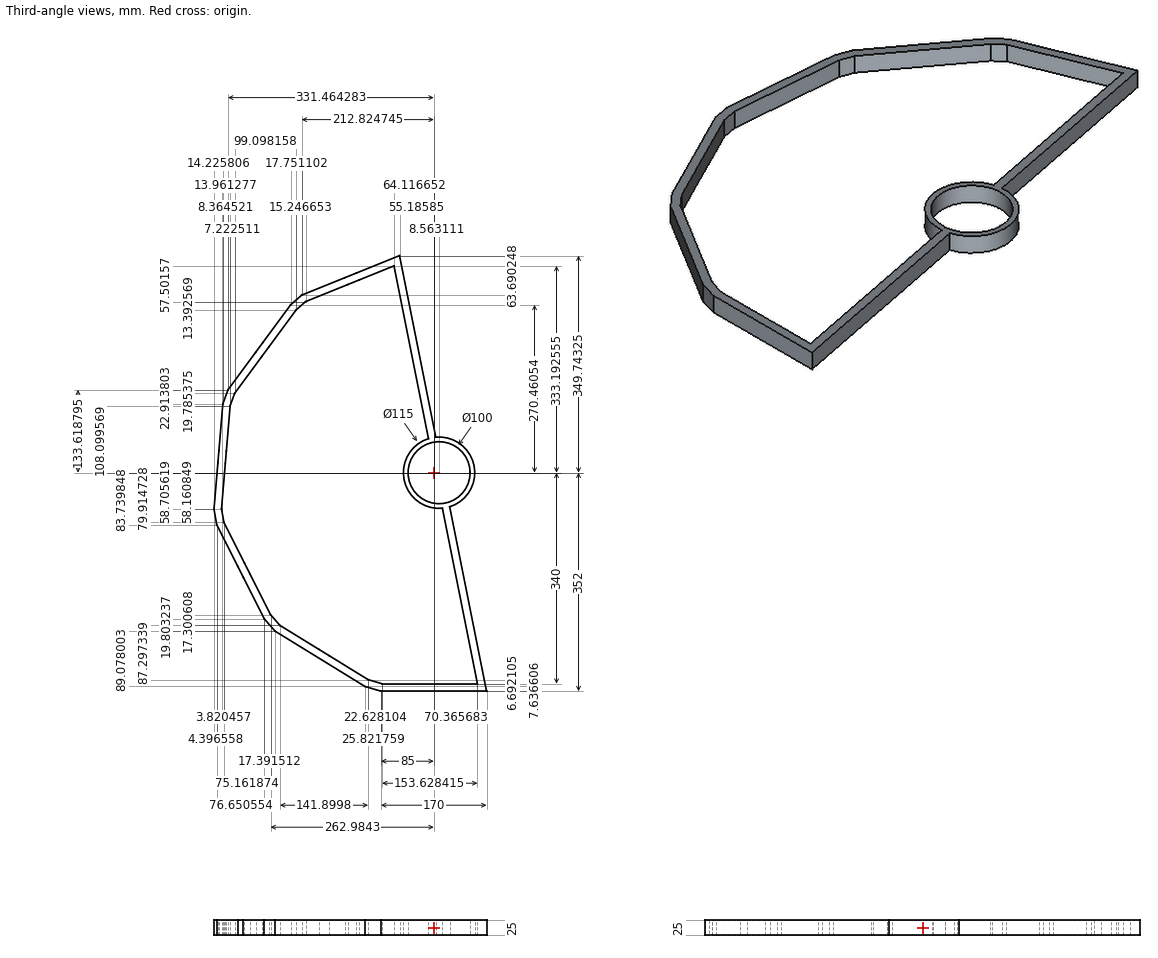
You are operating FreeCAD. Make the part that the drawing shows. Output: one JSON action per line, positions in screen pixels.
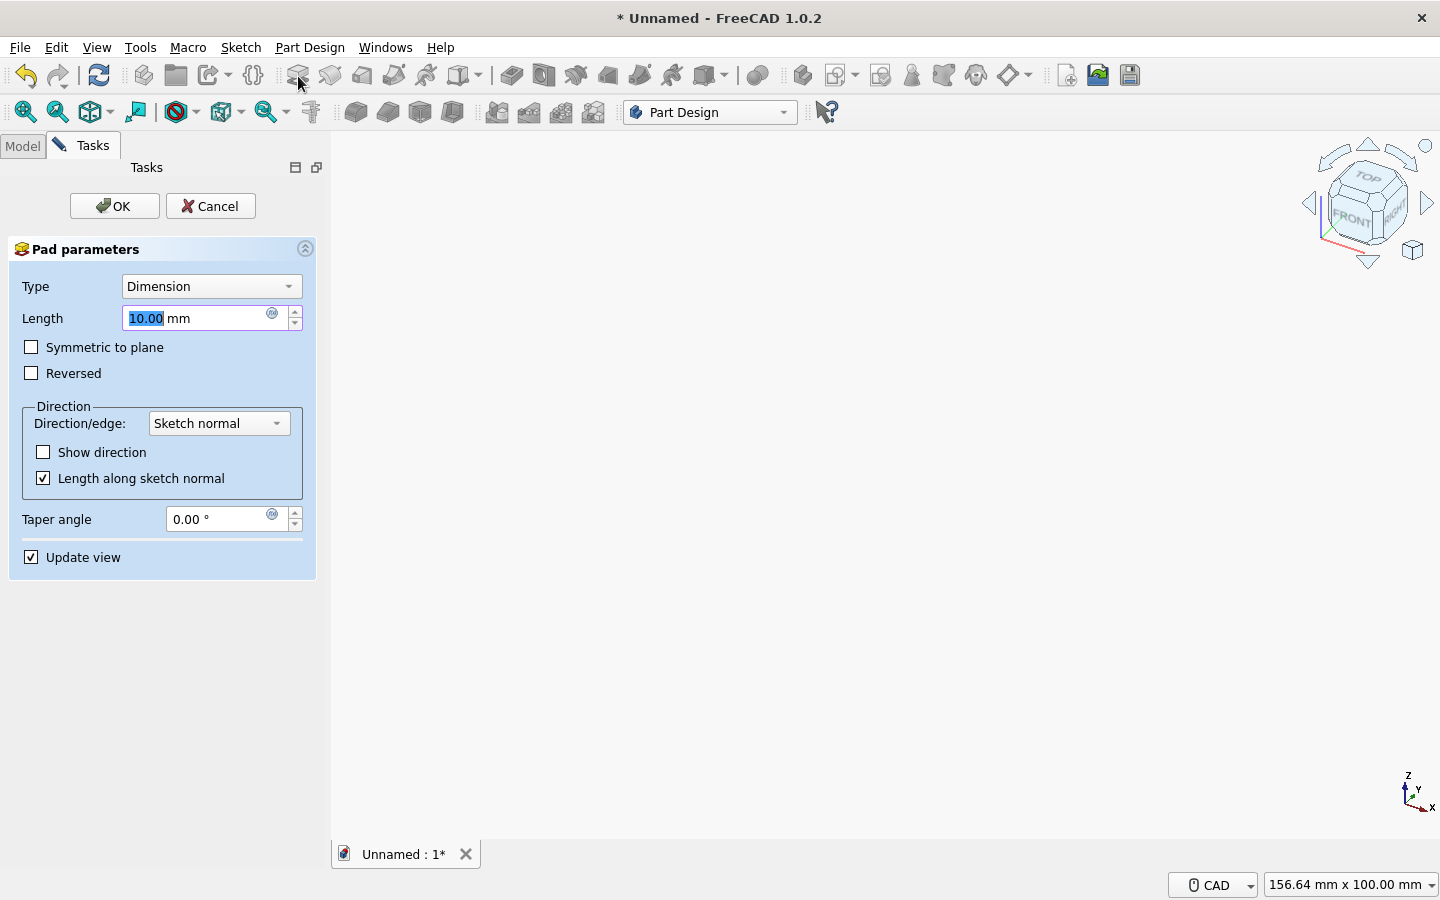
{"action": "type", "text": "25"}
{"action": "key", "text": "Tab"}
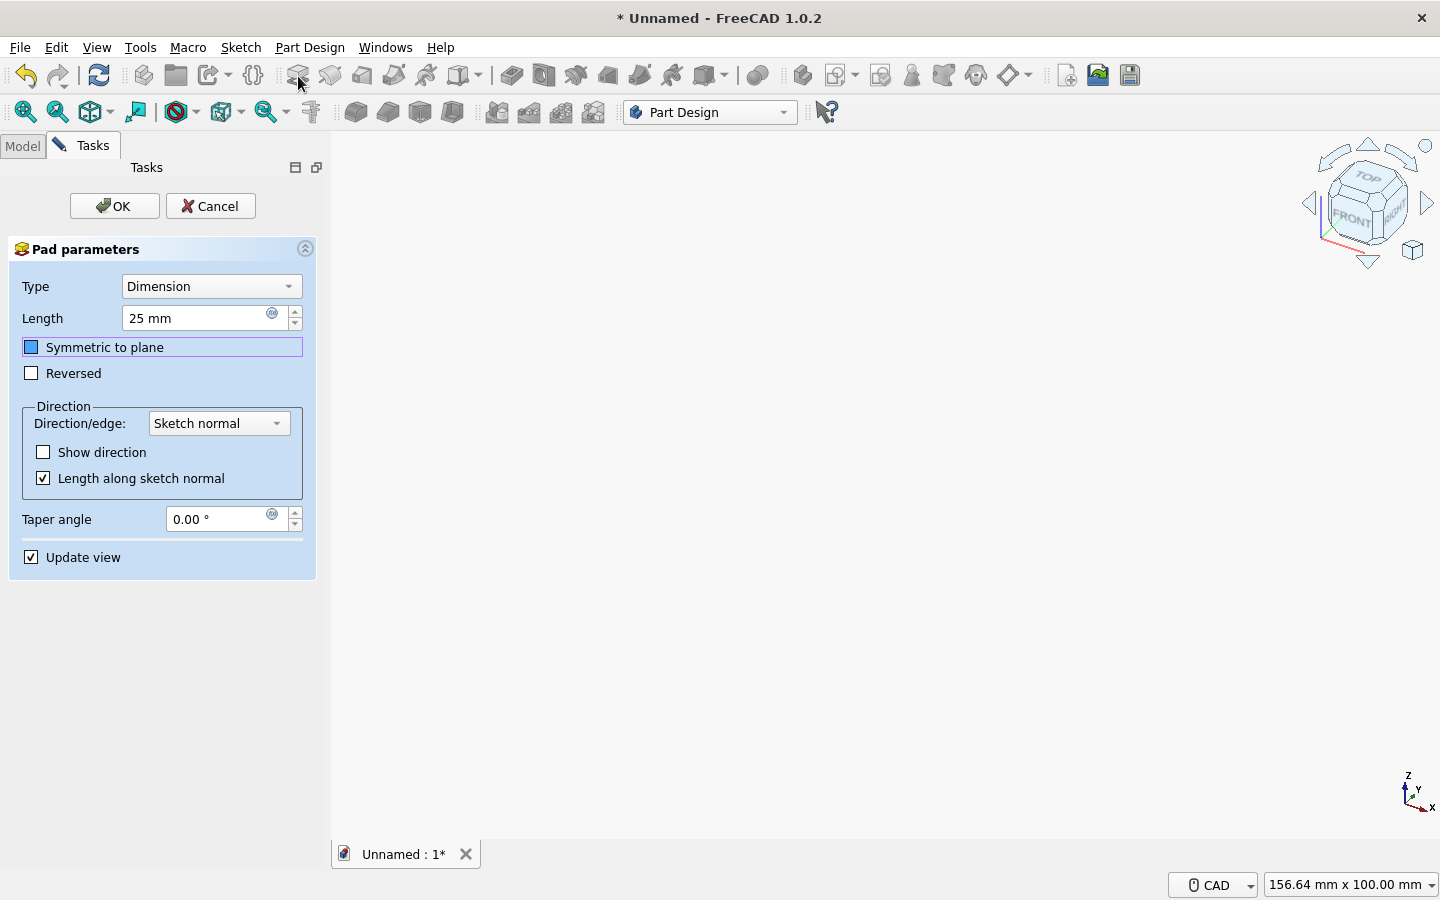
{"action": "left_click", "coordinate": [30, 347]}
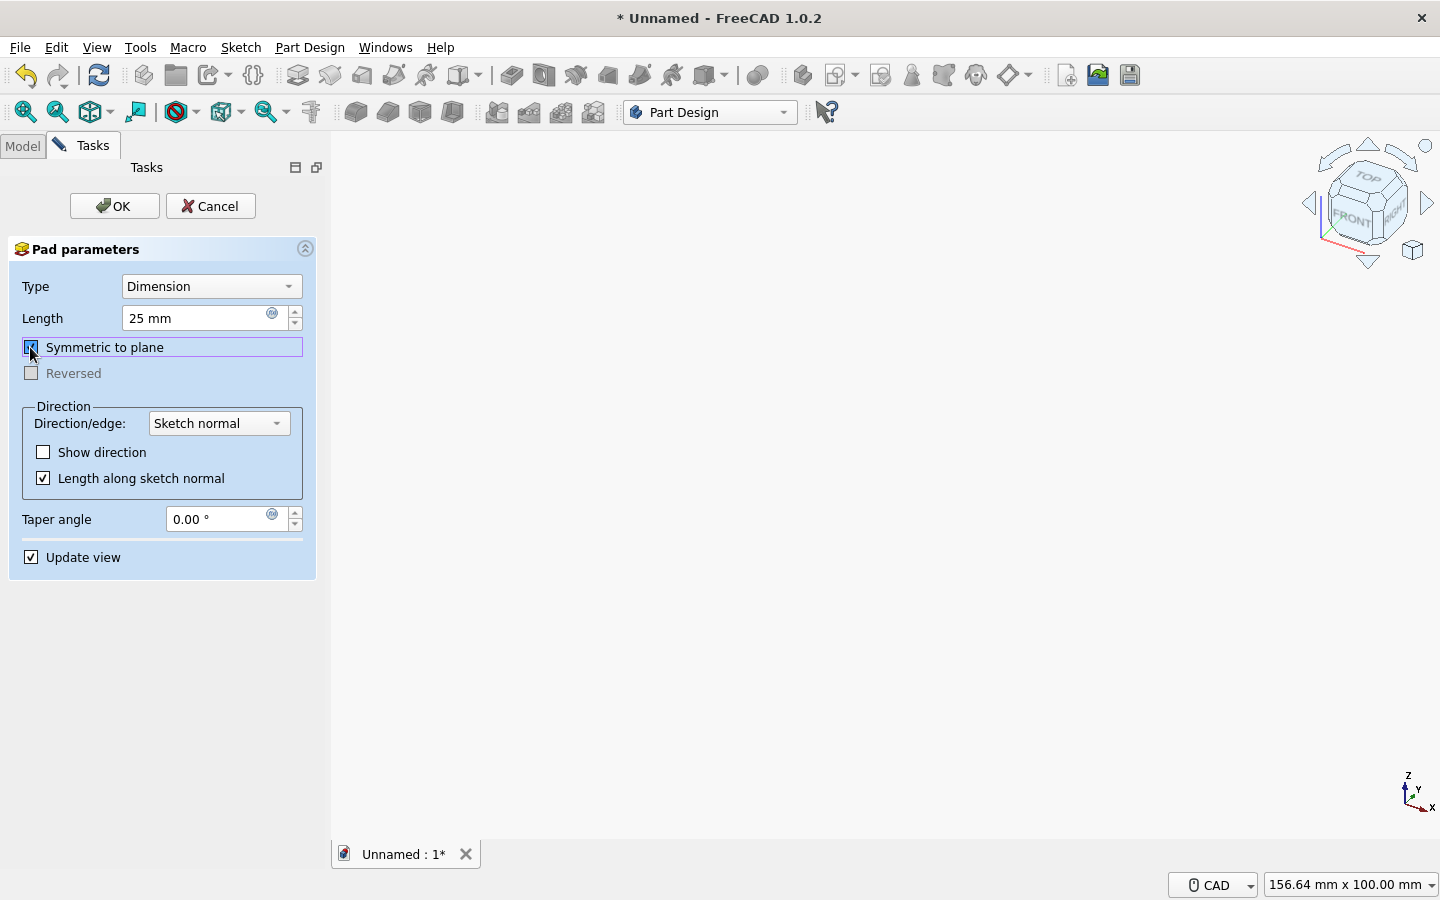
{"action": "left_click", "coordinate": [115, 206]}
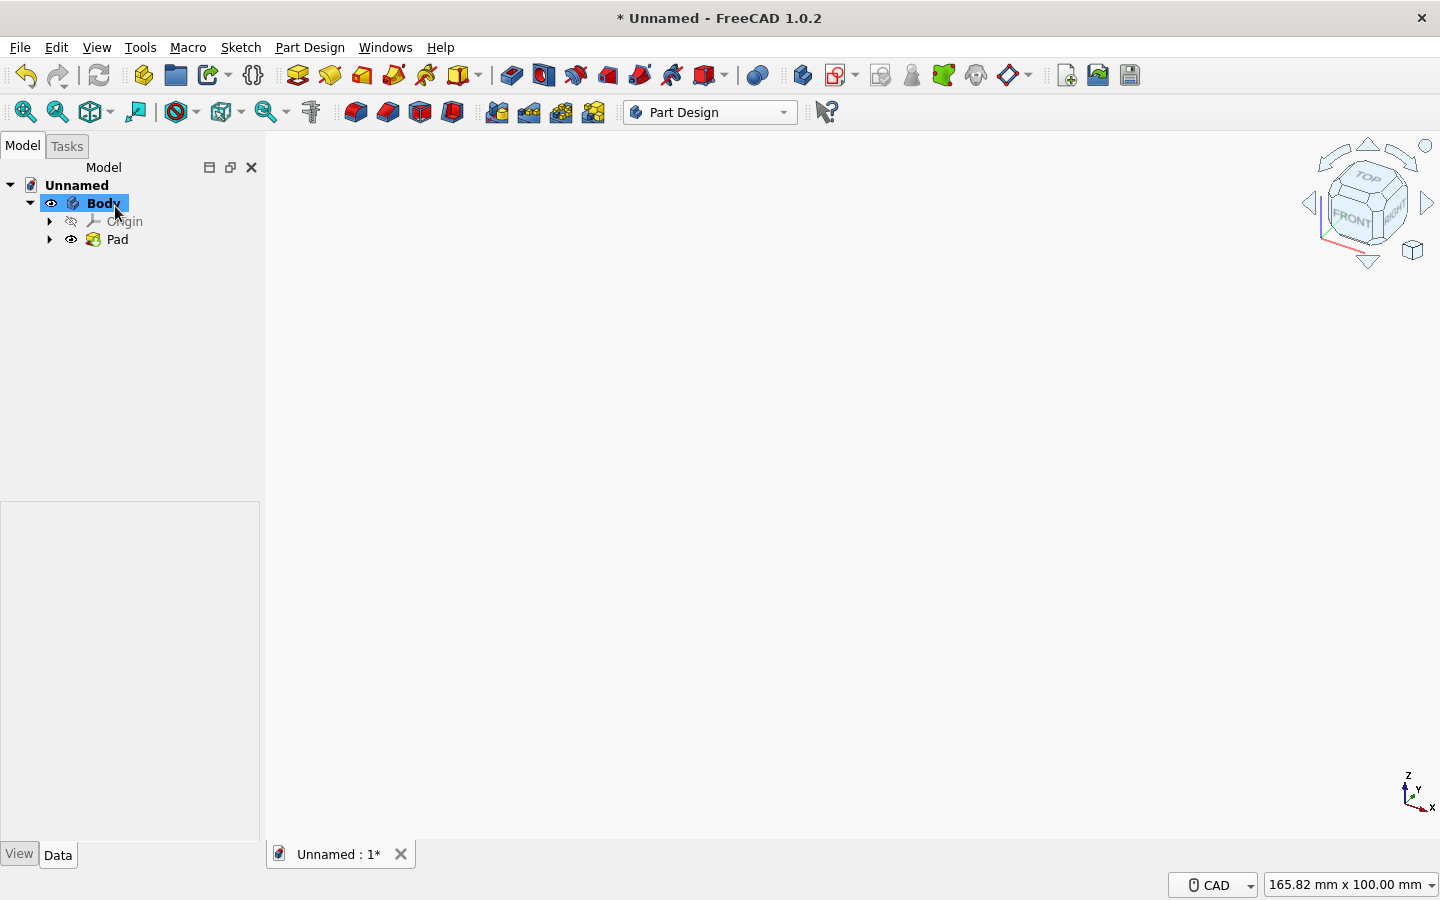
{"action": "left_click", "coordinate": [26, 112]}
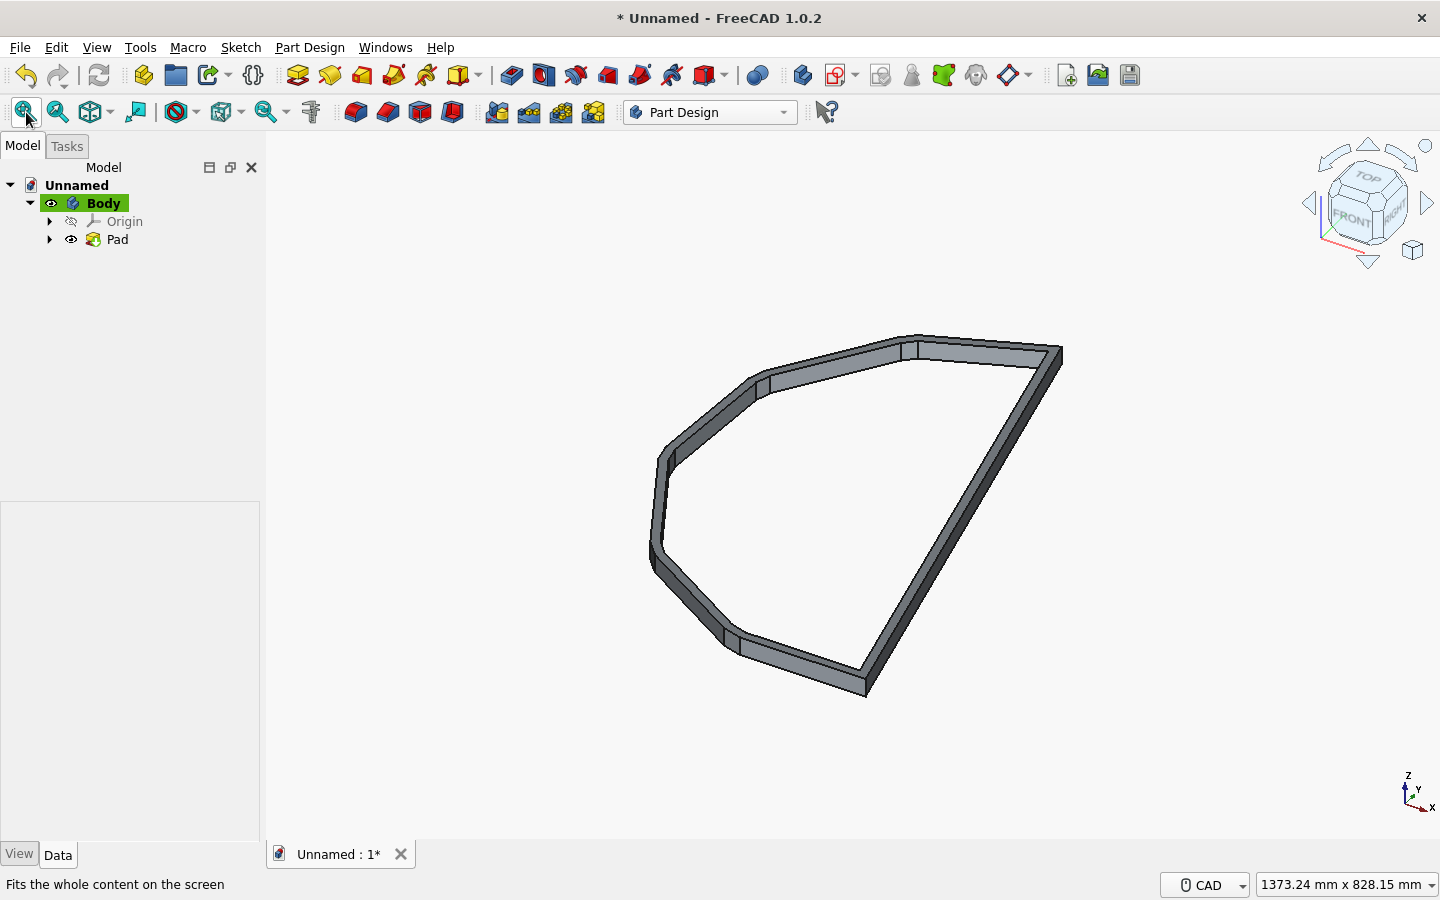
{"action": "scroll", "coordinate": [734, 627], "scroll_direction": "up", "scroll_amount": 7}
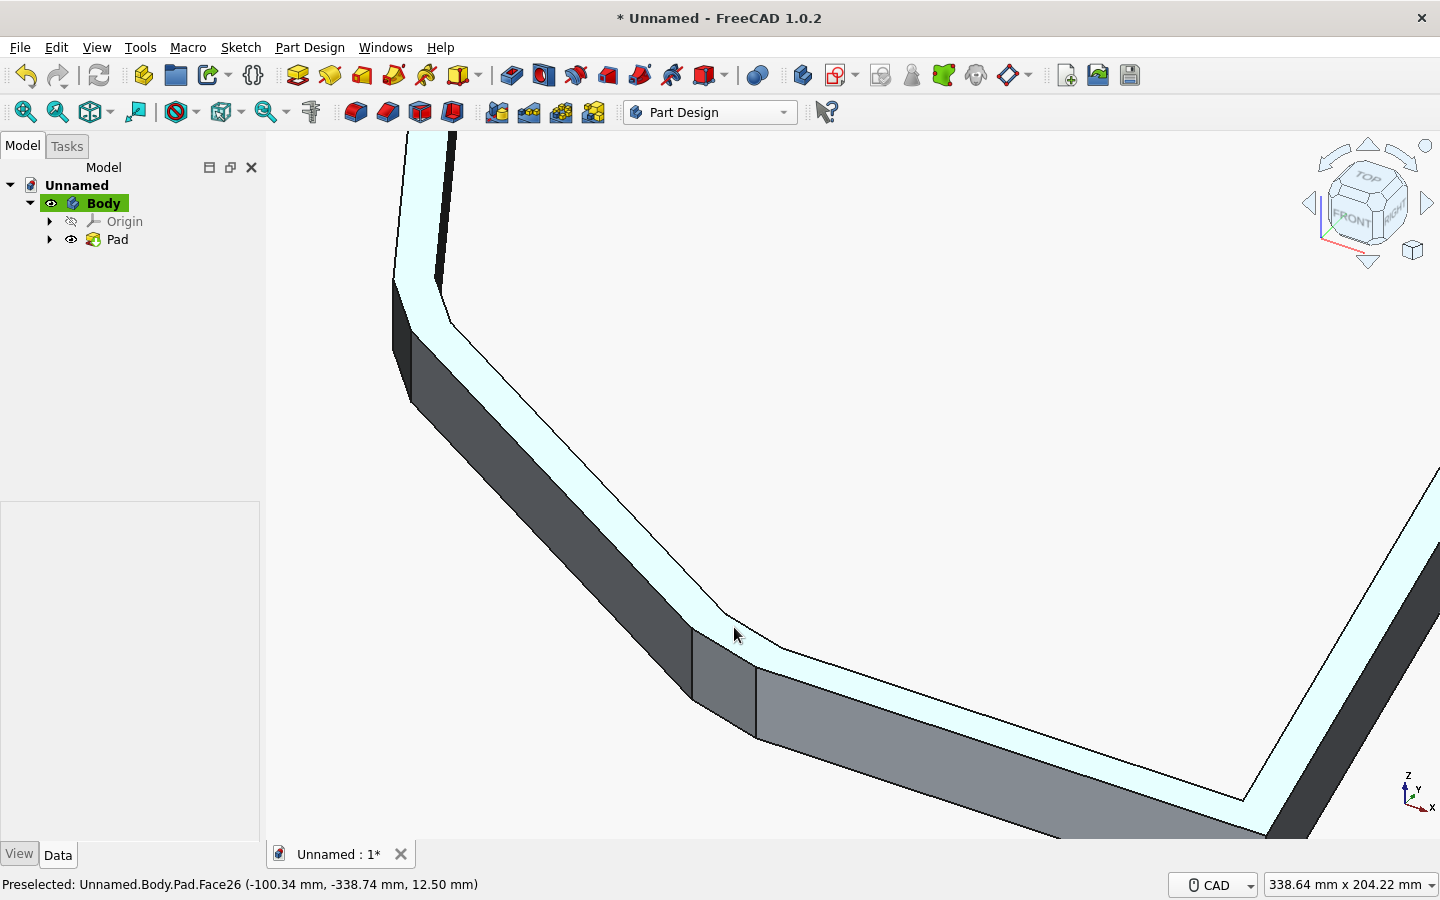
{"action": "left_click", "coordinate": [733, 629]}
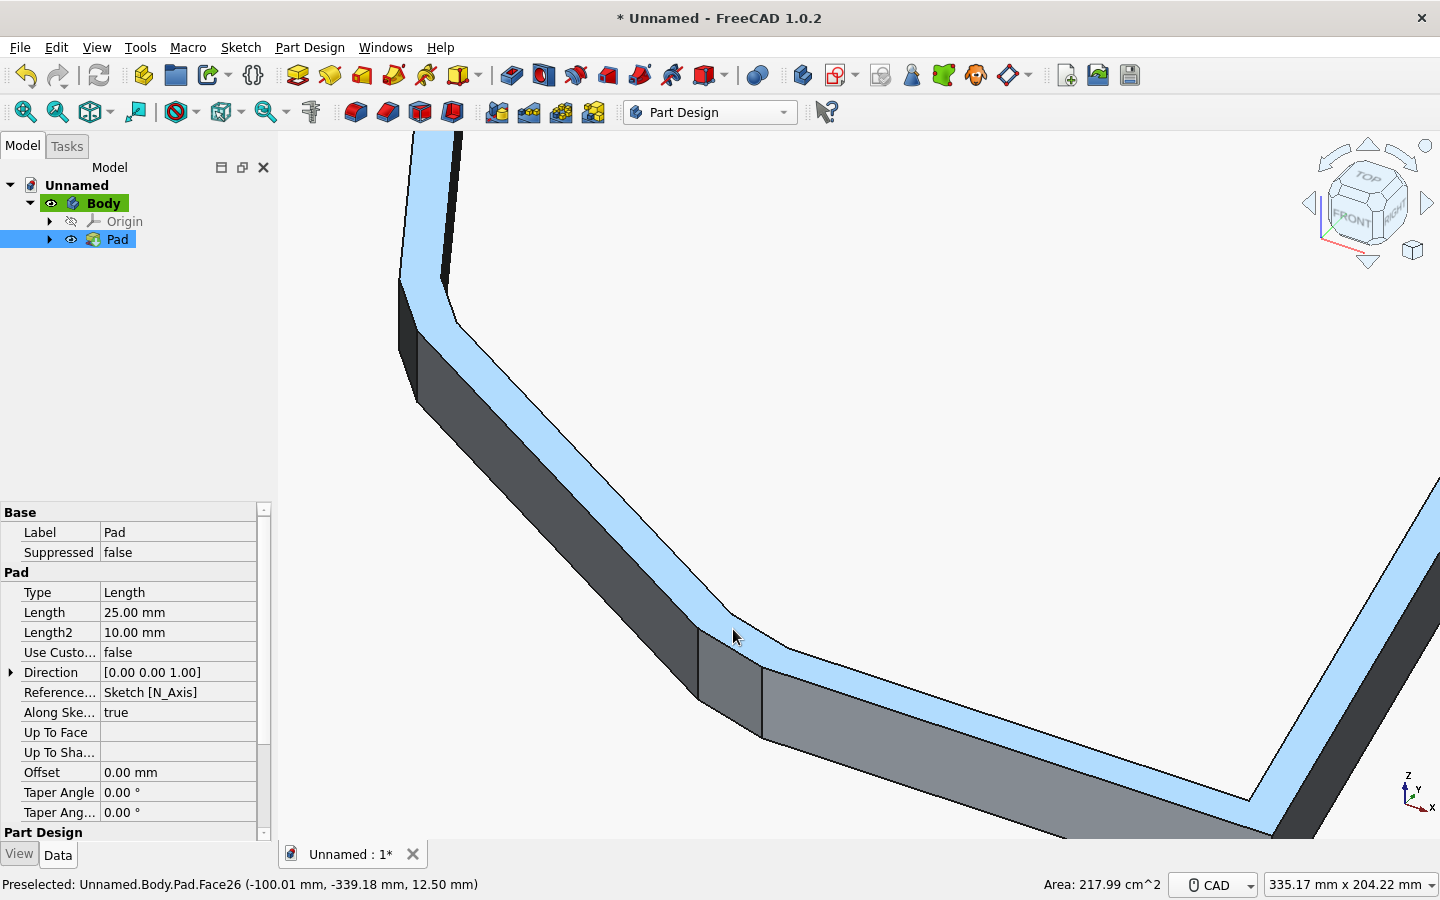
{"action": "left_click", "coordinate": [836, 76]}